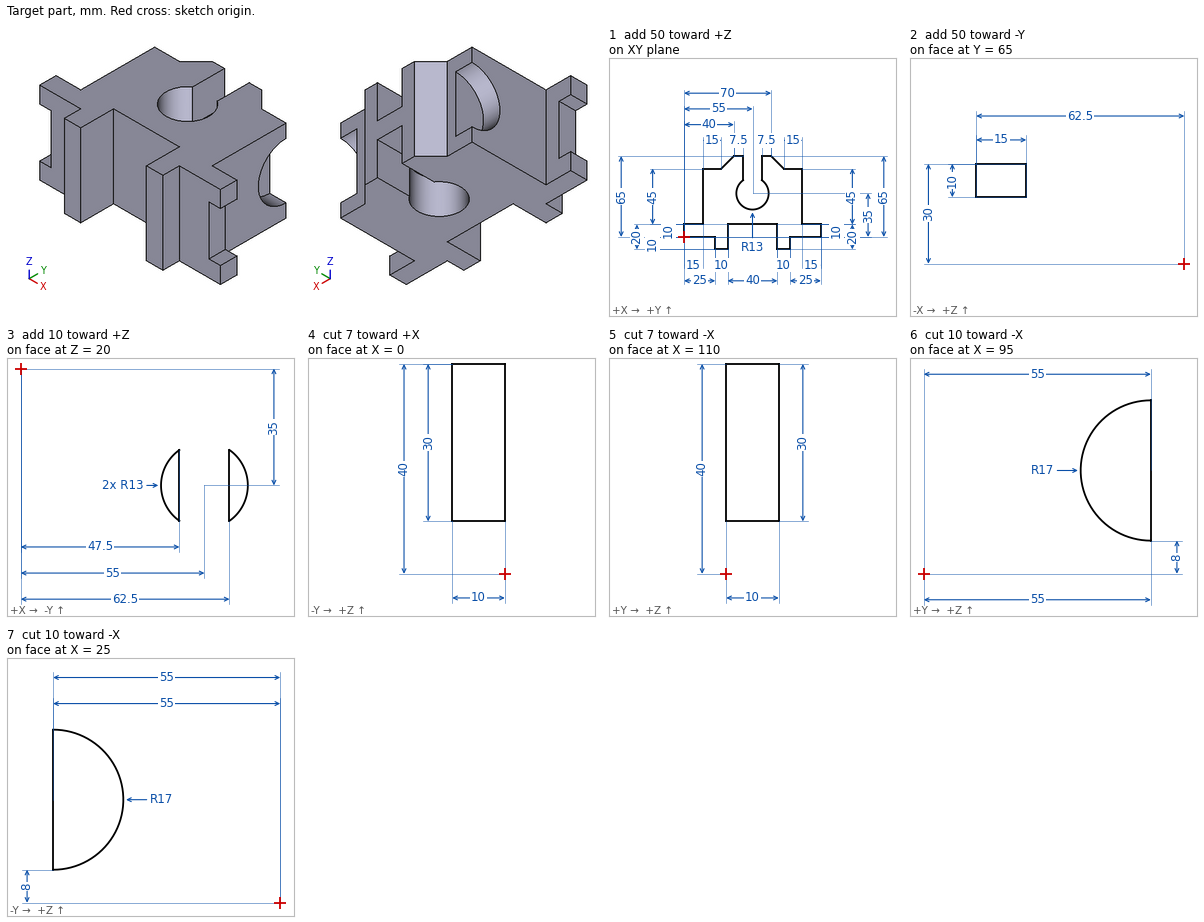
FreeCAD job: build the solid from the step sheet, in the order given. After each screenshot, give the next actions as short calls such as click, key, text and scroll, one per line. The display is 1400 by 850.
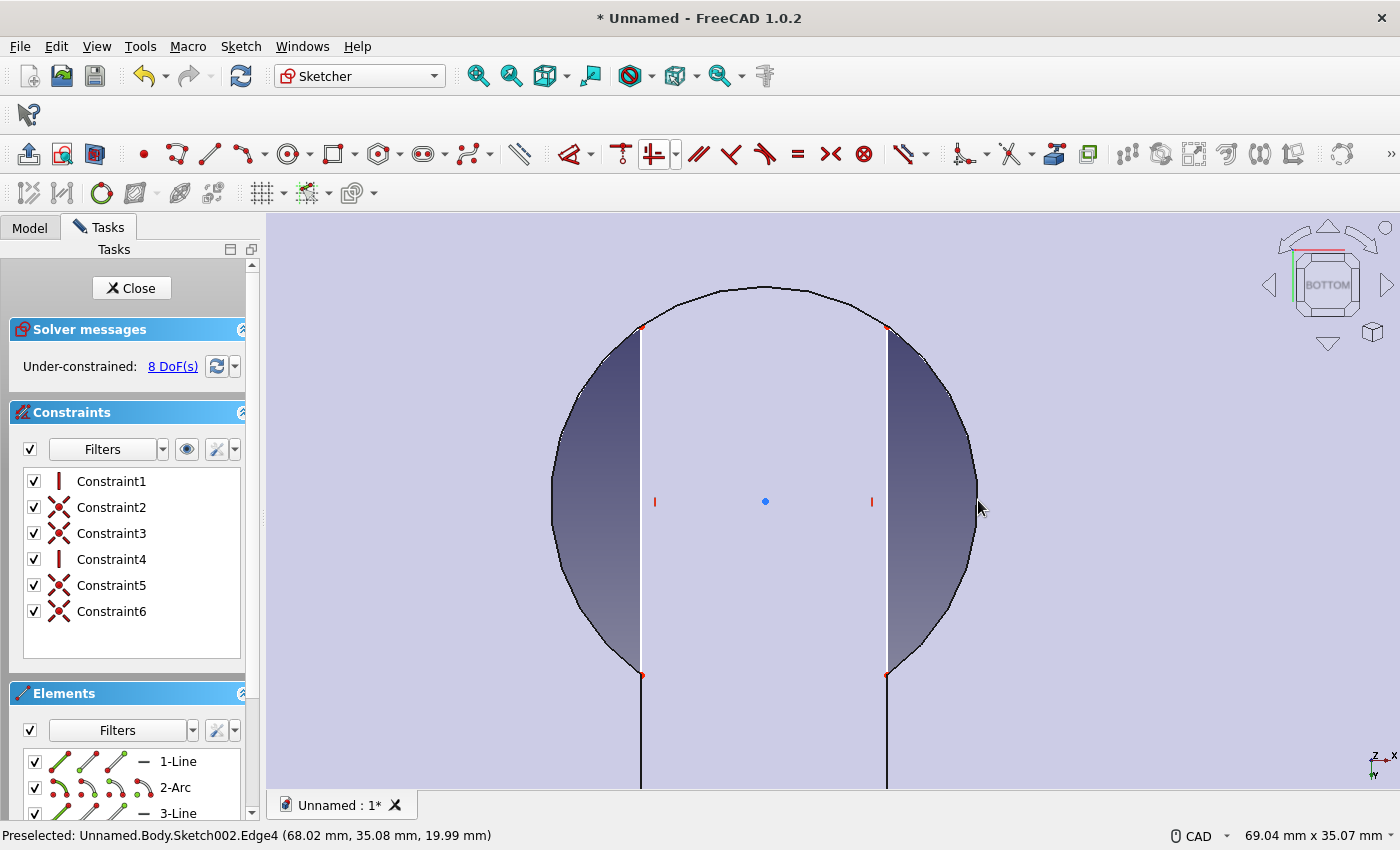
click(566, 422)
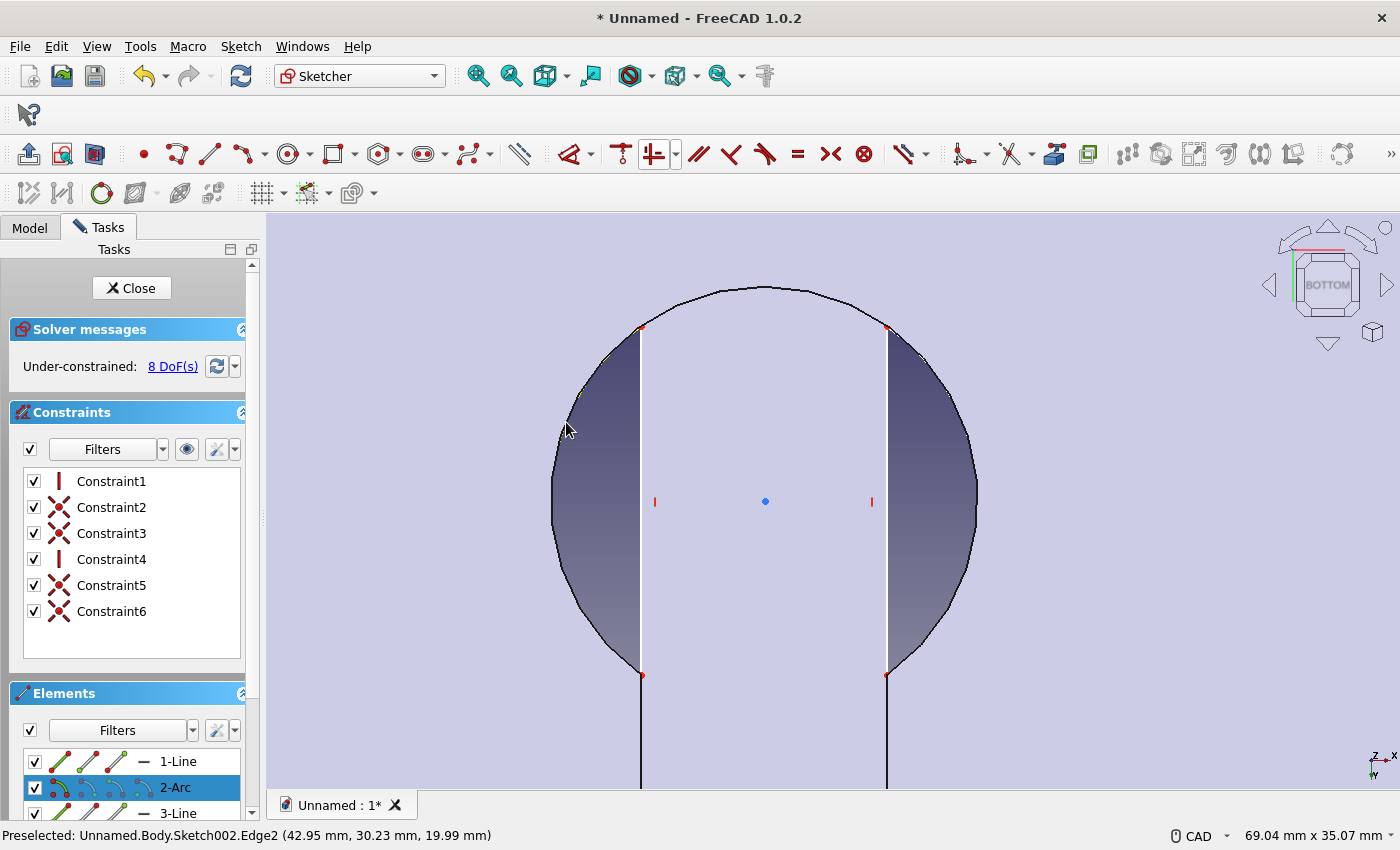
click(962, 581)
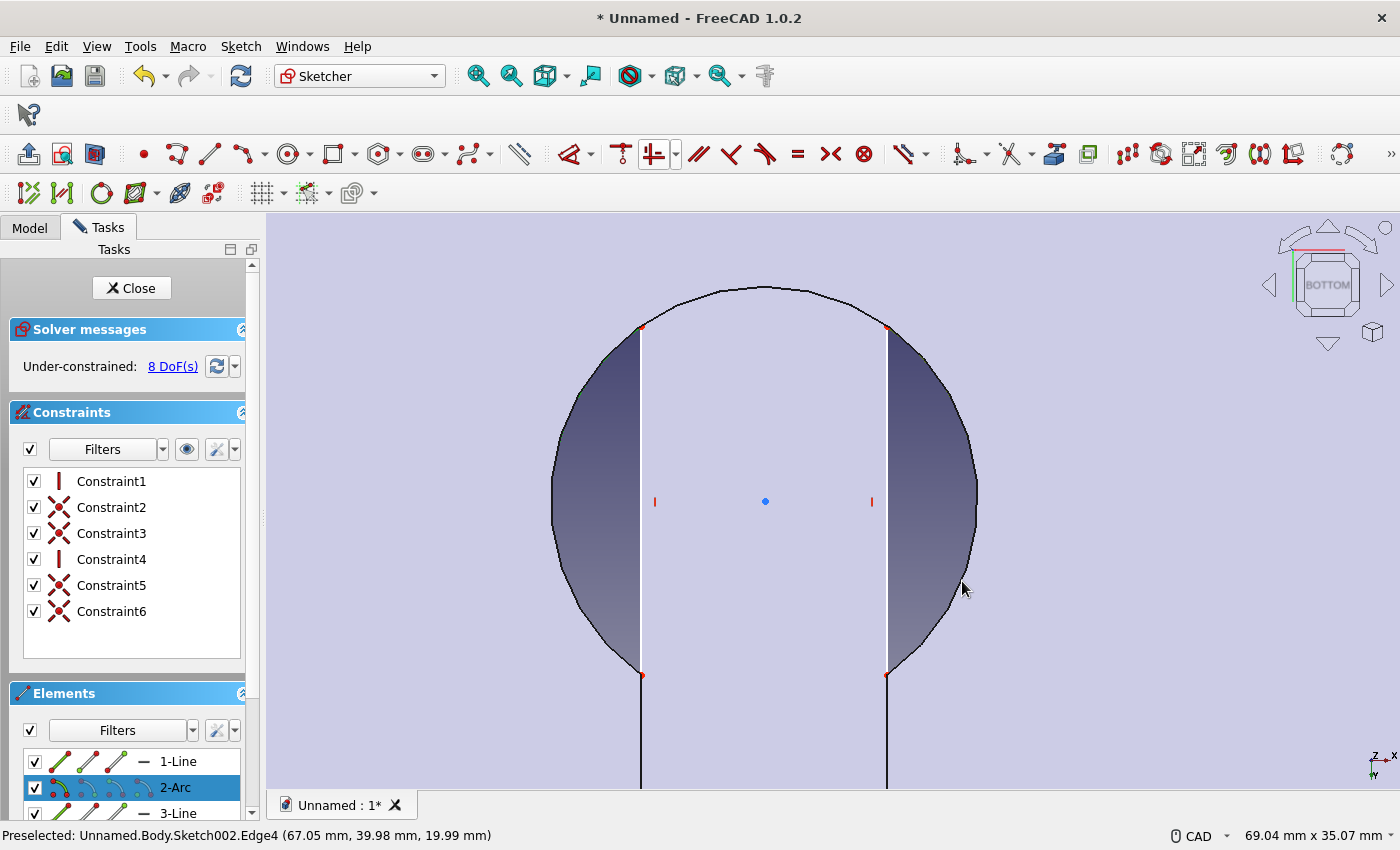
click(621, 154)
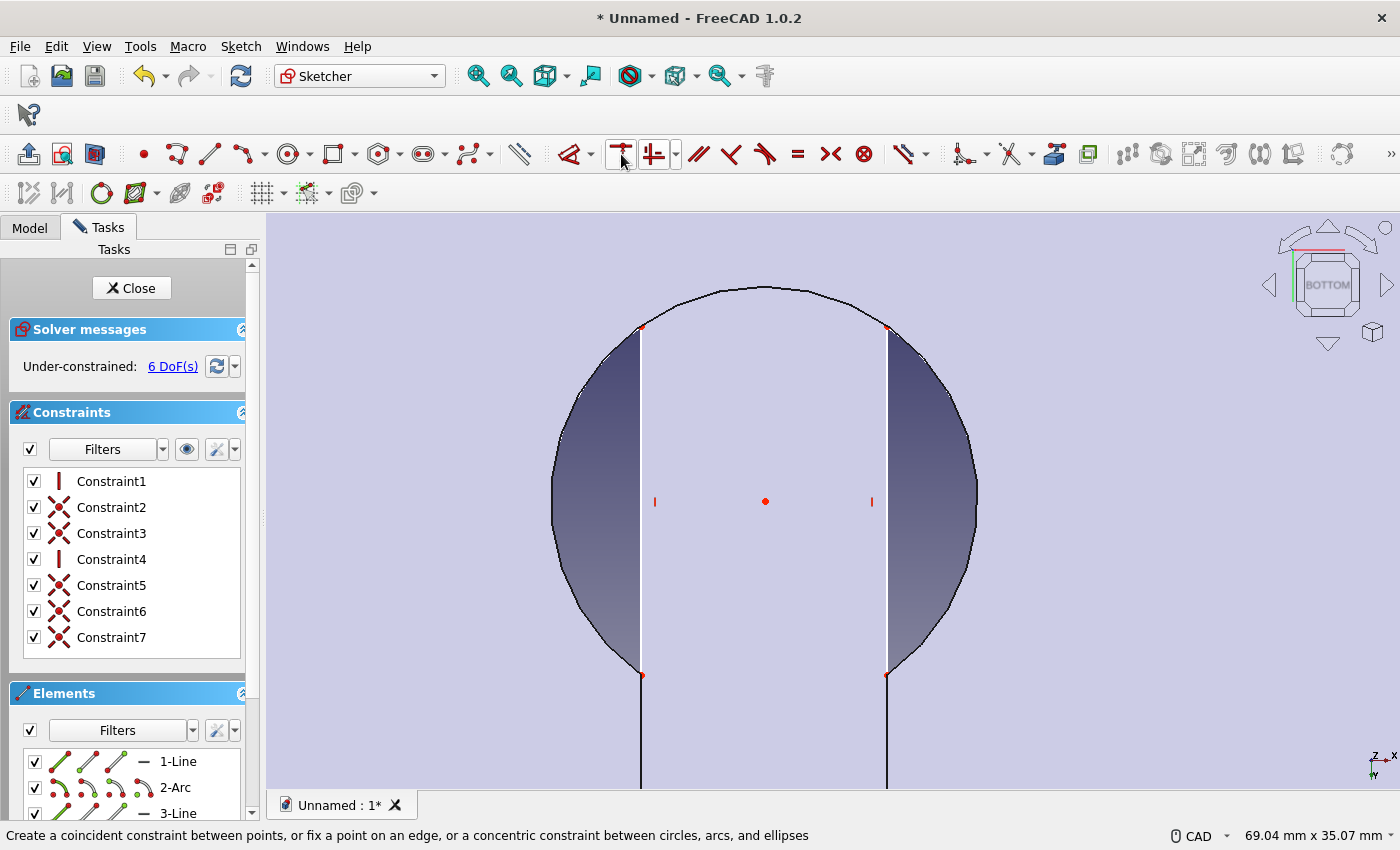
click(566, 422)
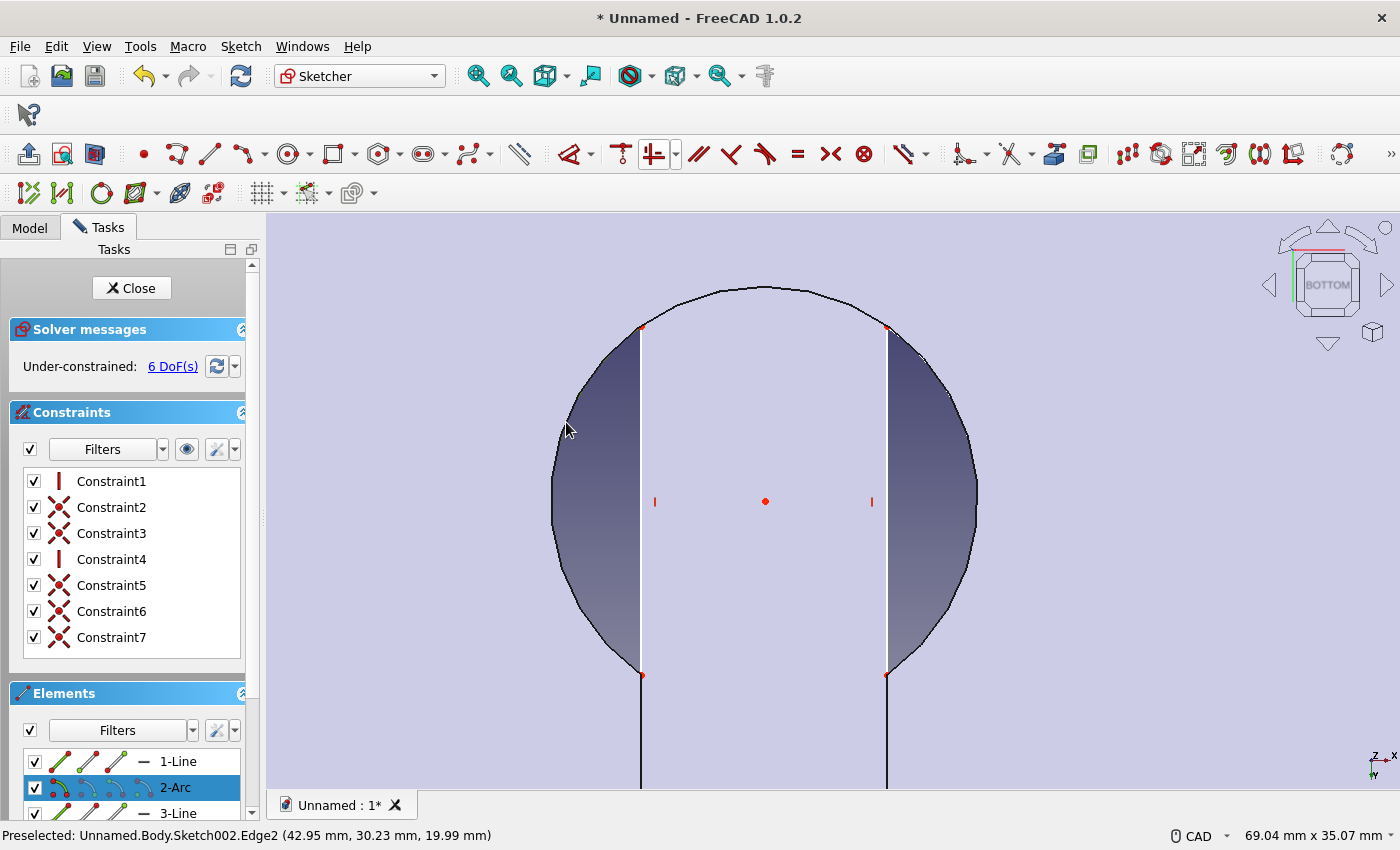
click(962, 581)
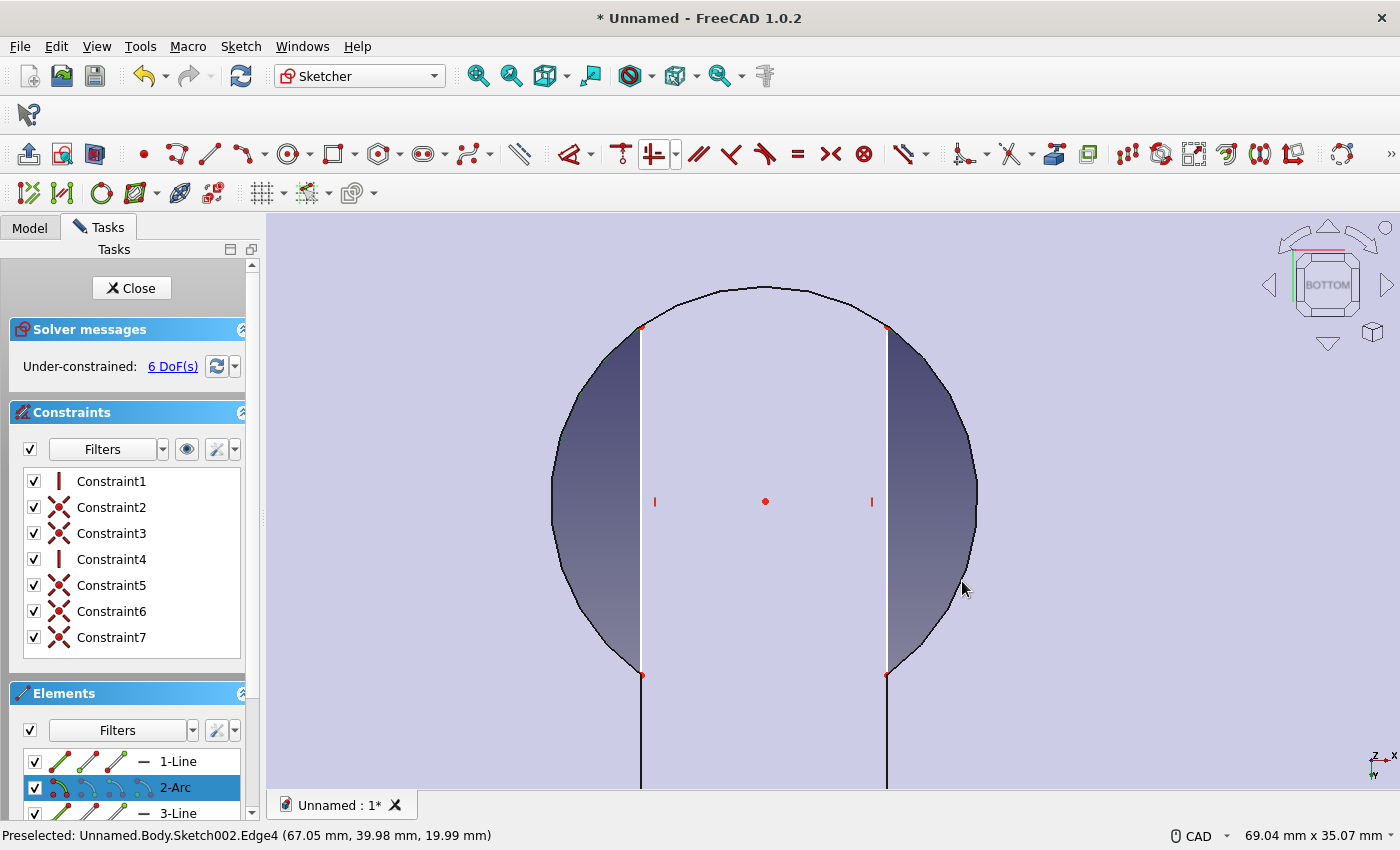
click(798, 154)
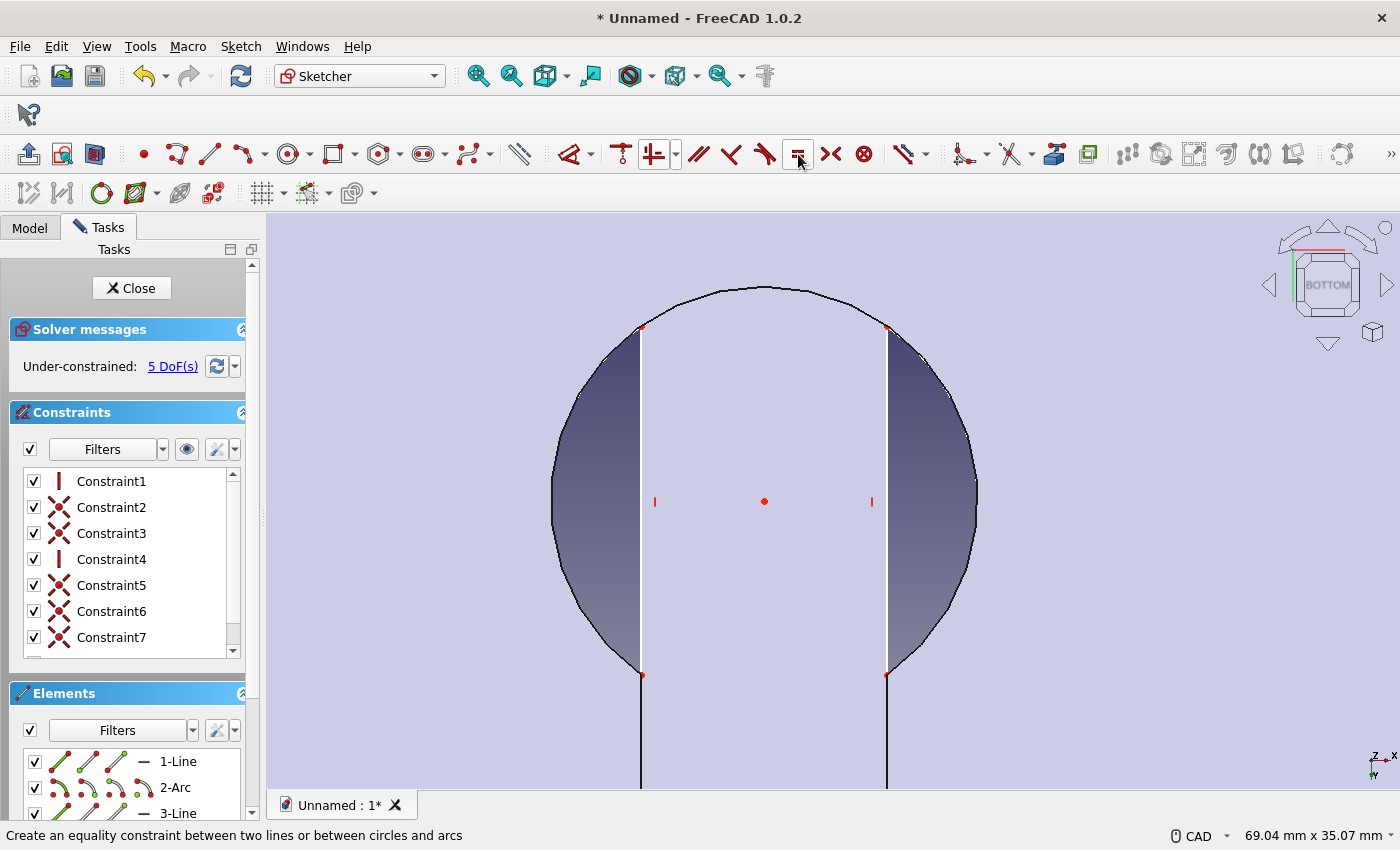
click(568, 154)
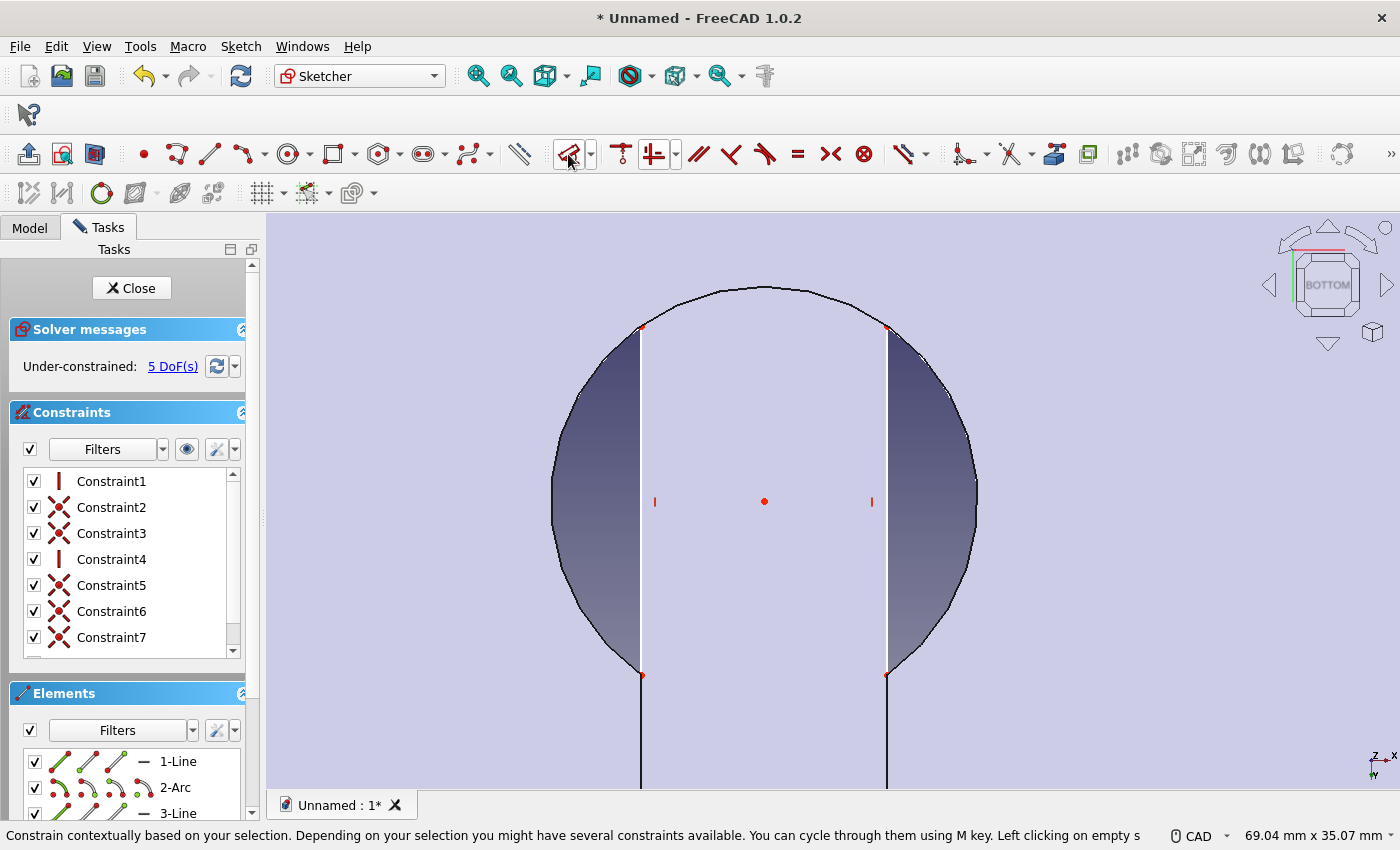
click(566, 422)
click(536, 410)